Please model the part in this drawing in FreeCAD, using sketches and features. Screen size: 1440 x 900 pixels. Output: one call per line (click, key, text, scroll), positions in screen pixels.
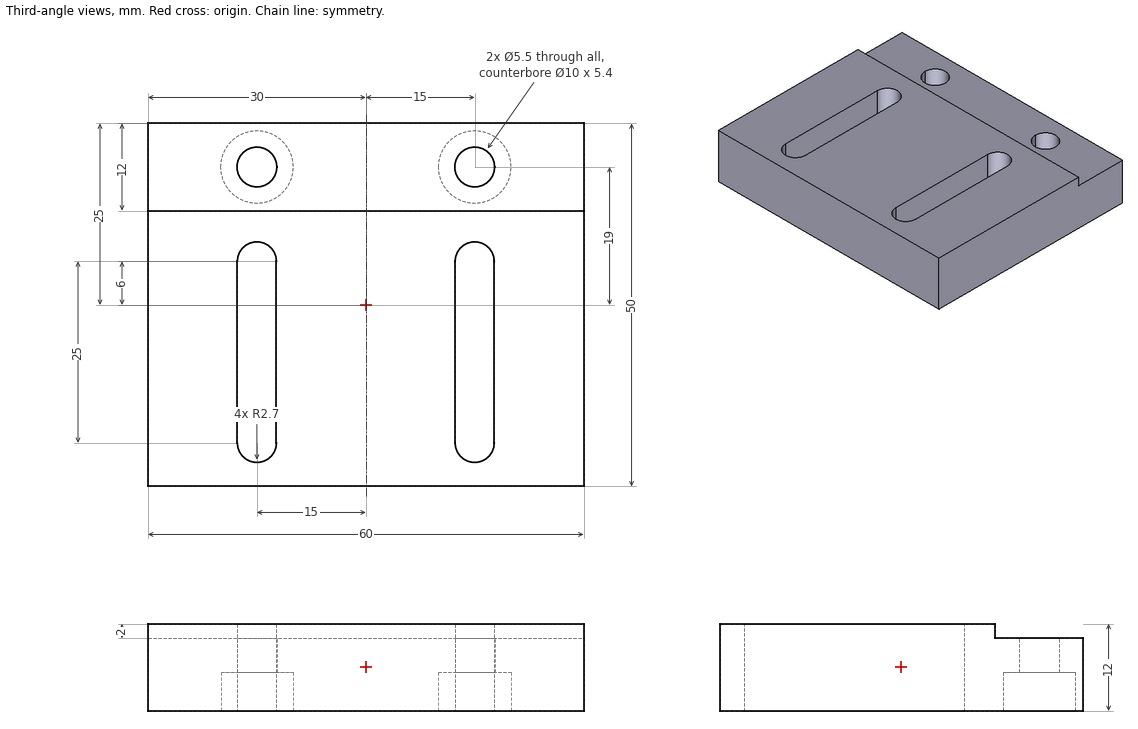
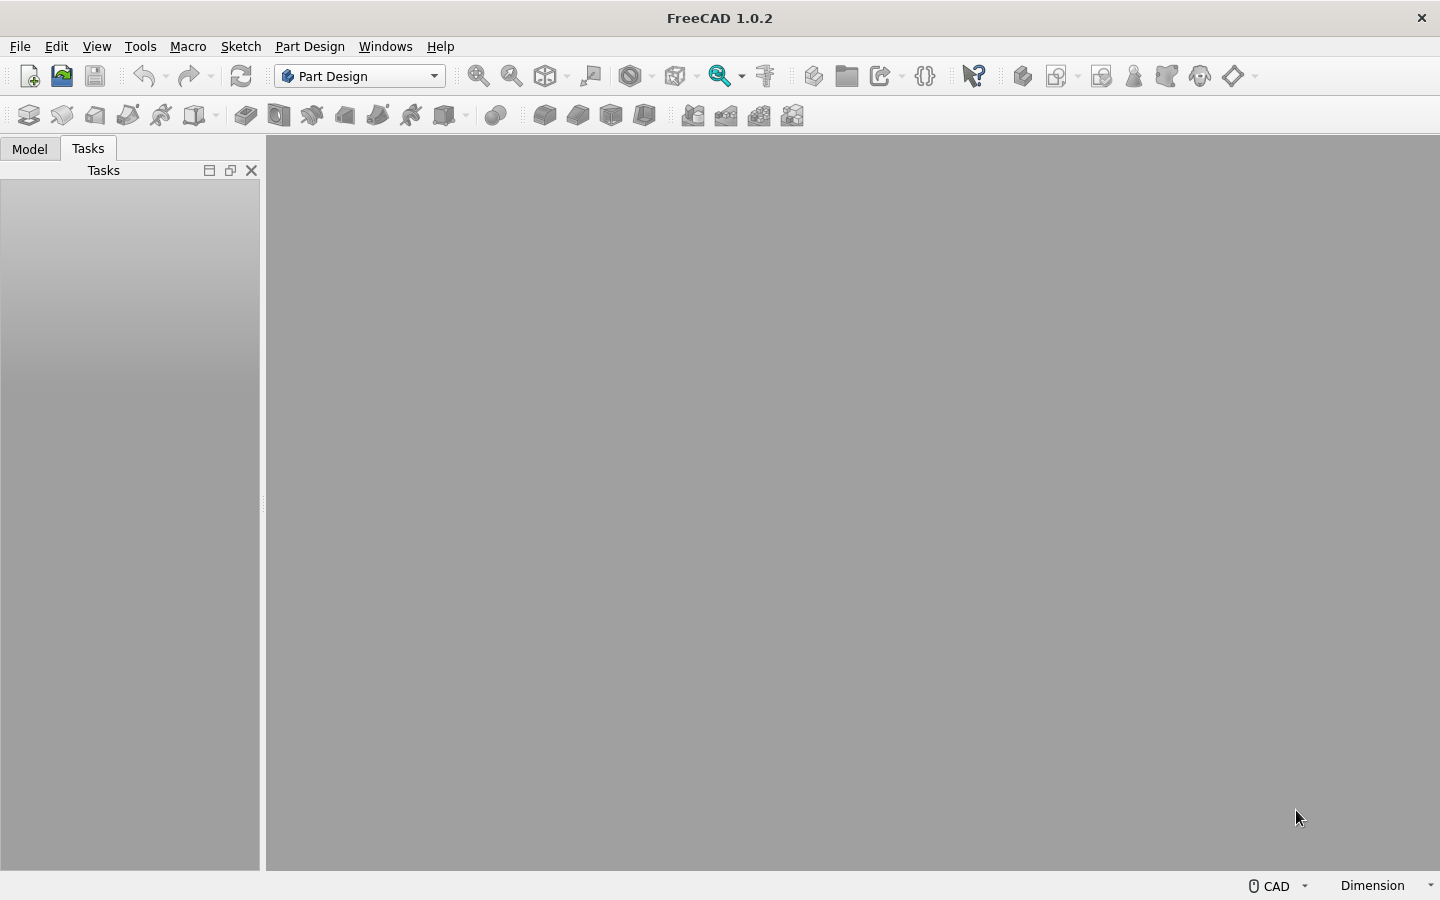
key(ctrl+n)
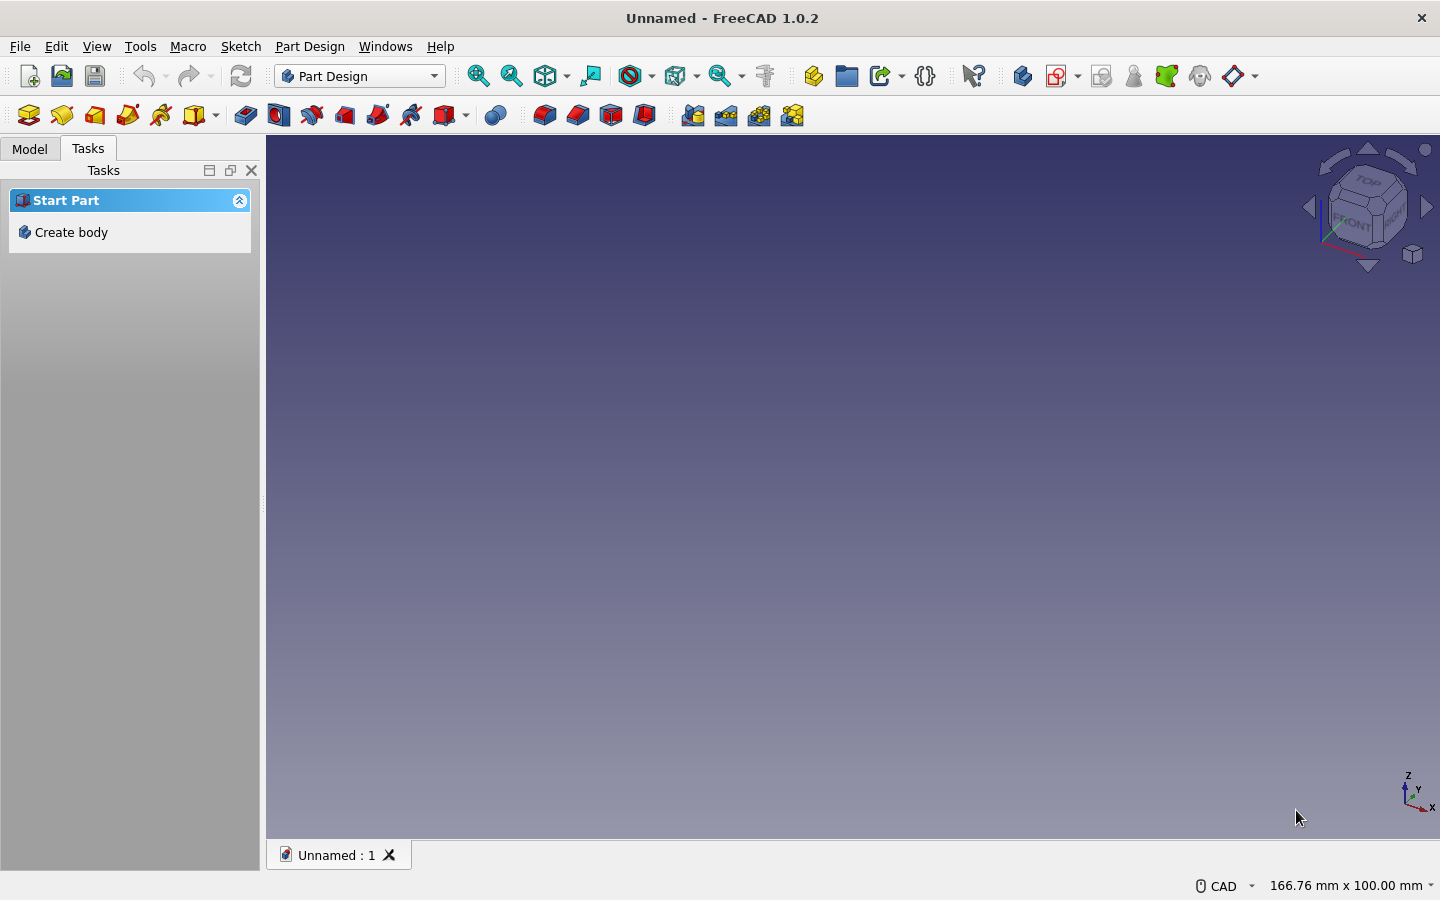
click(1056, 76)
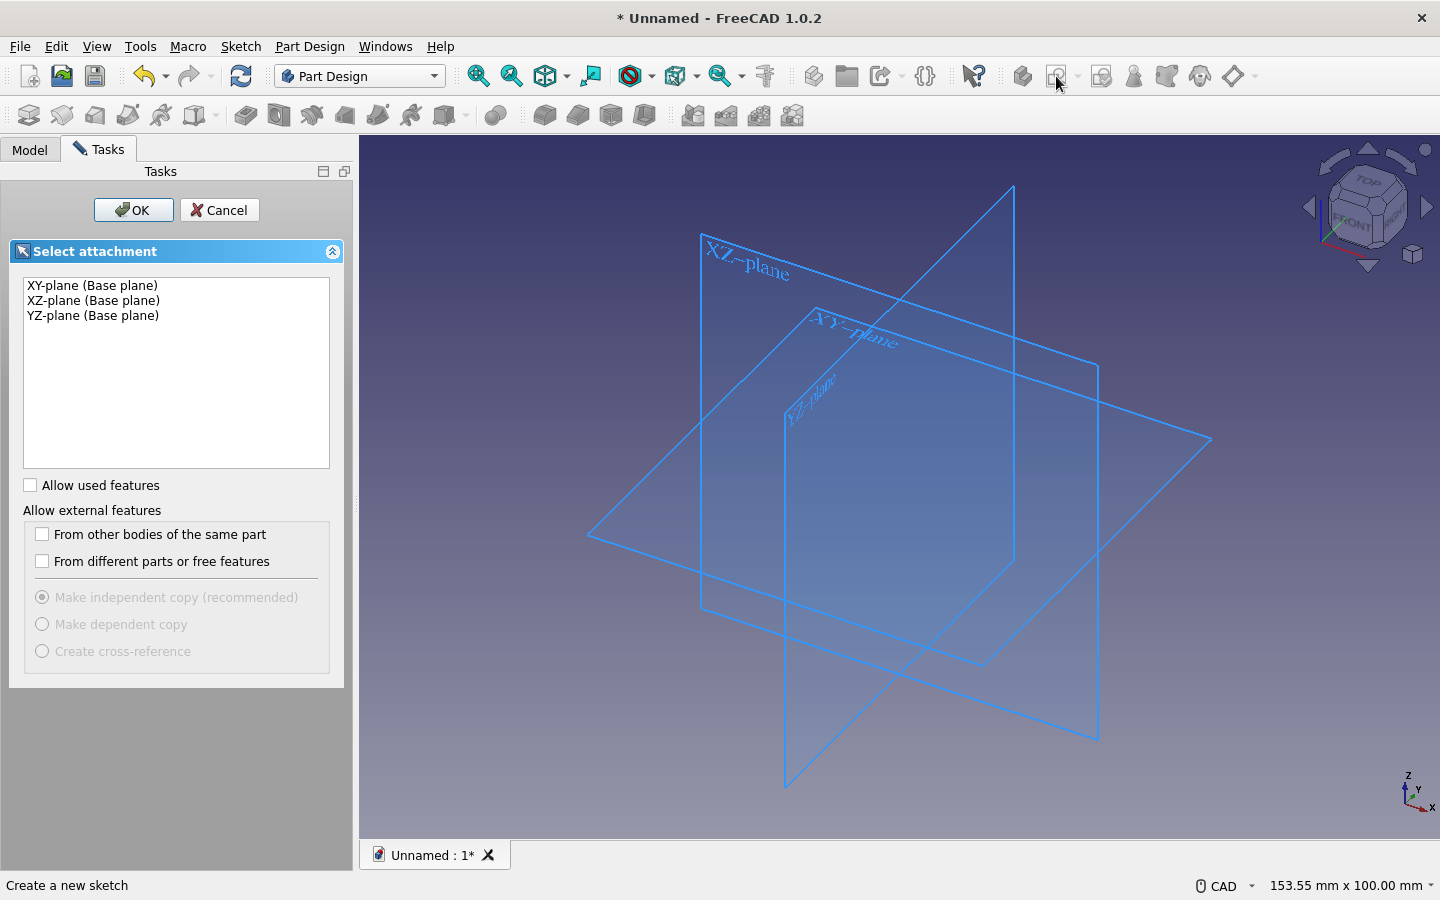
click(84, 286)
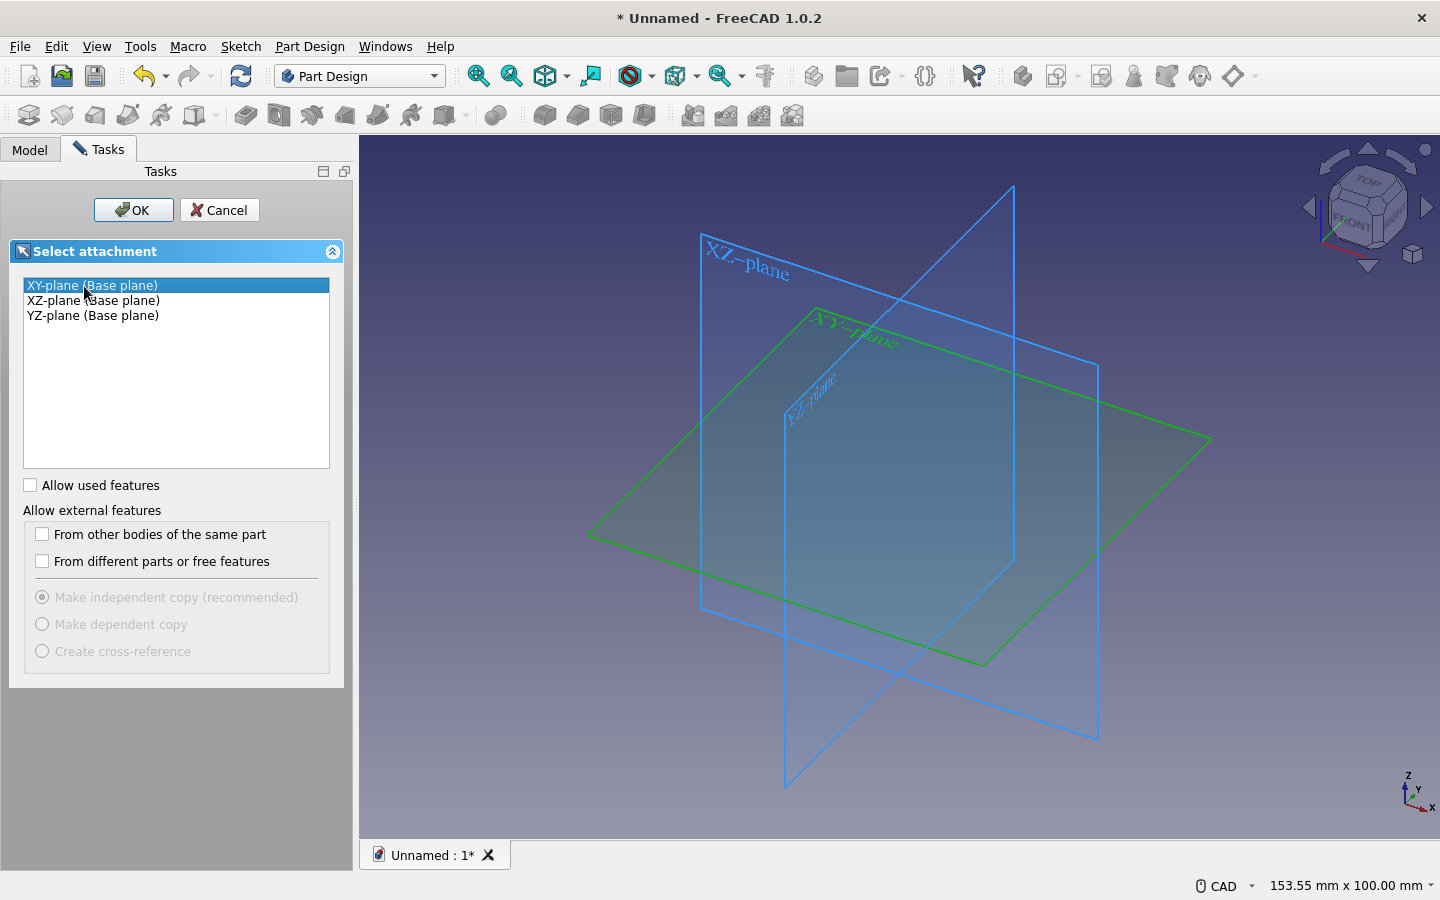
click(134, 210)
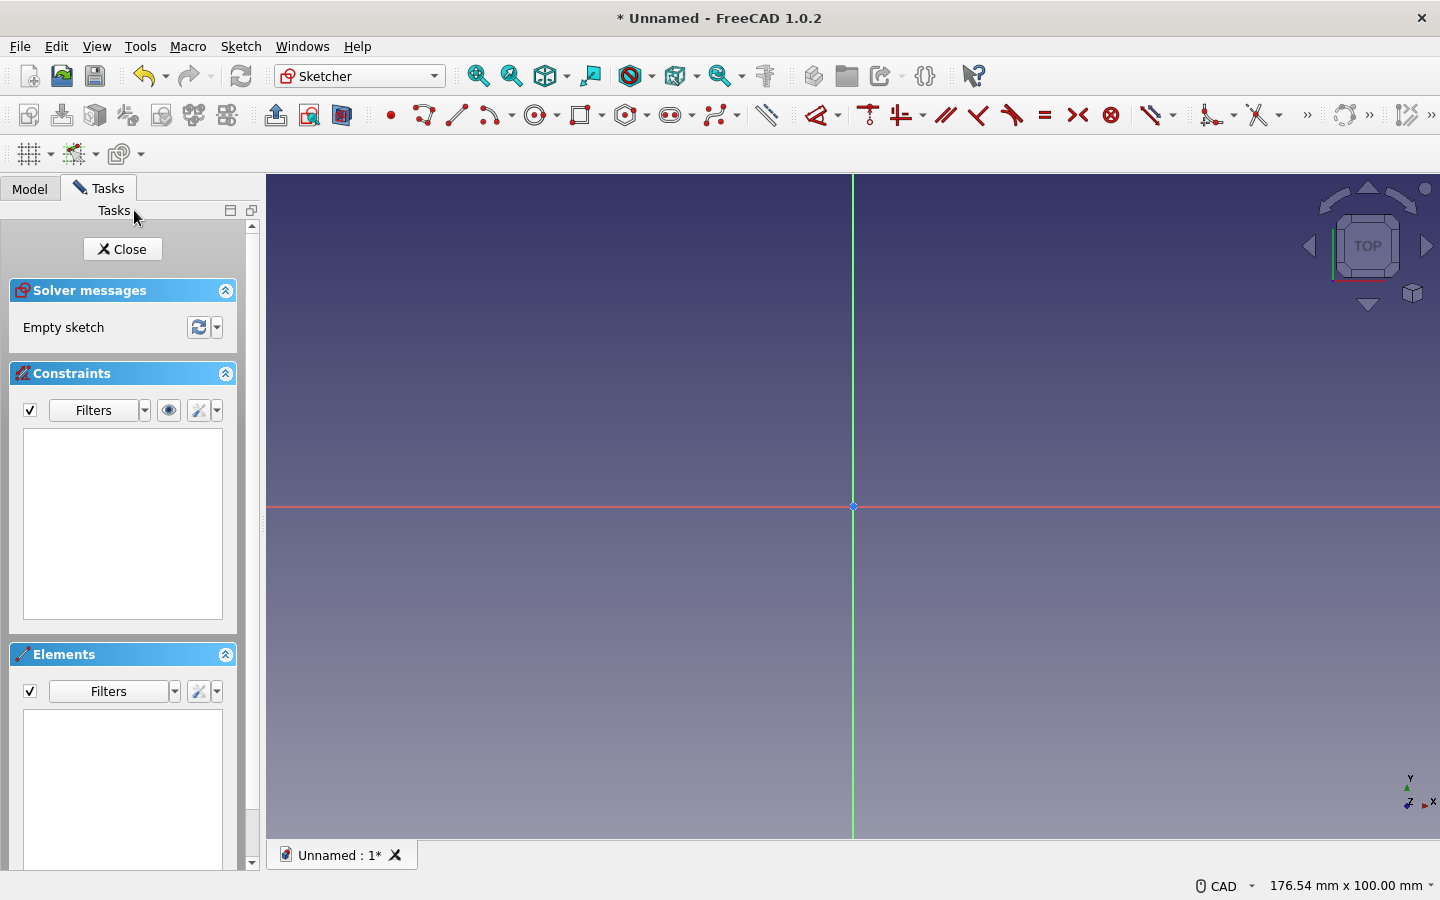
key(g)
key(v)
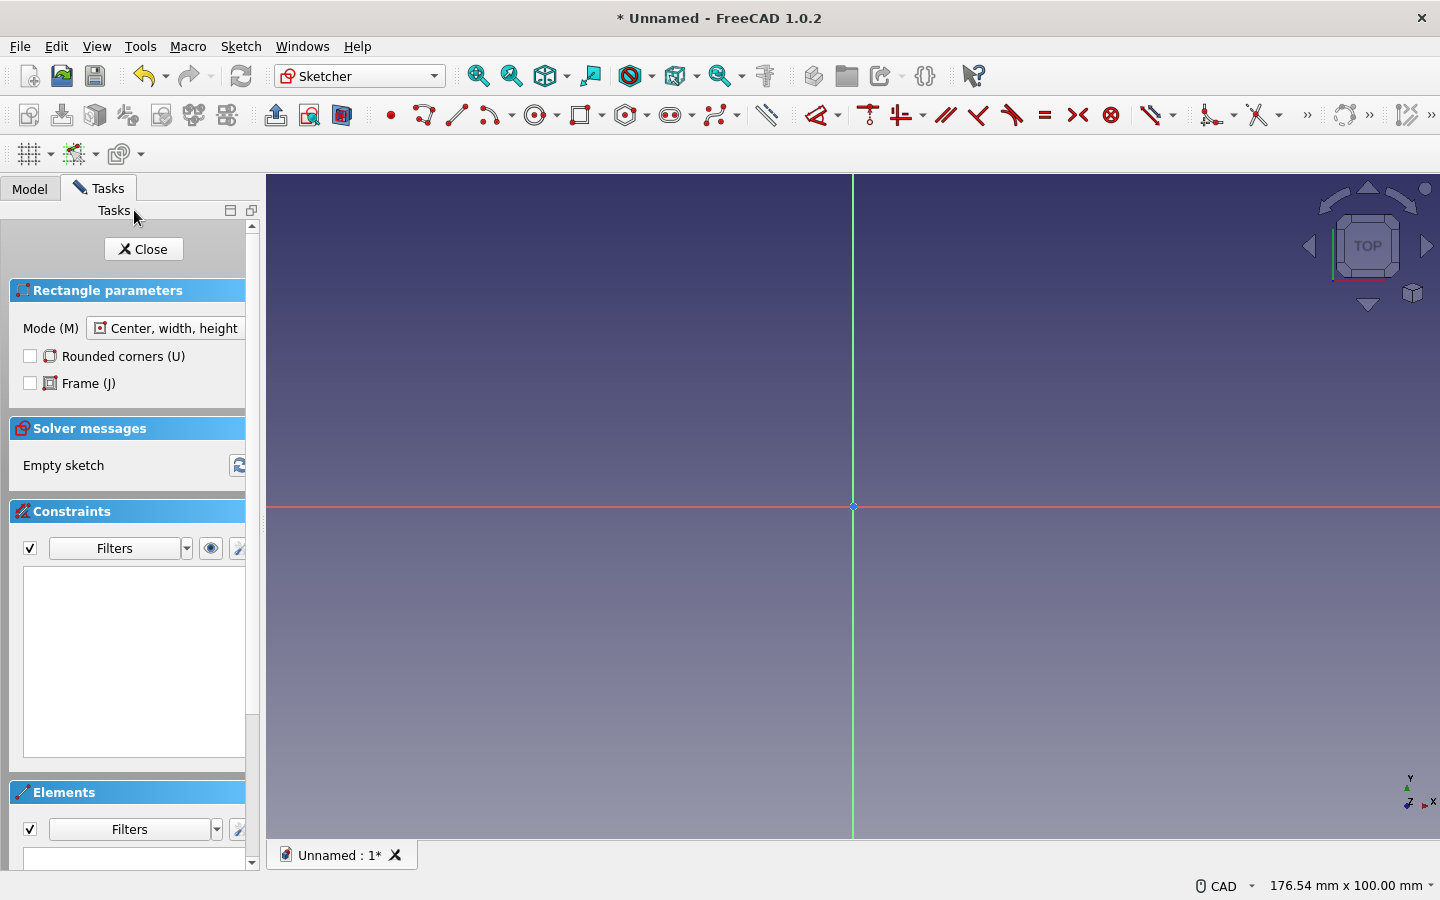
click(853, 506)
click(1052, 340)
key(Escape)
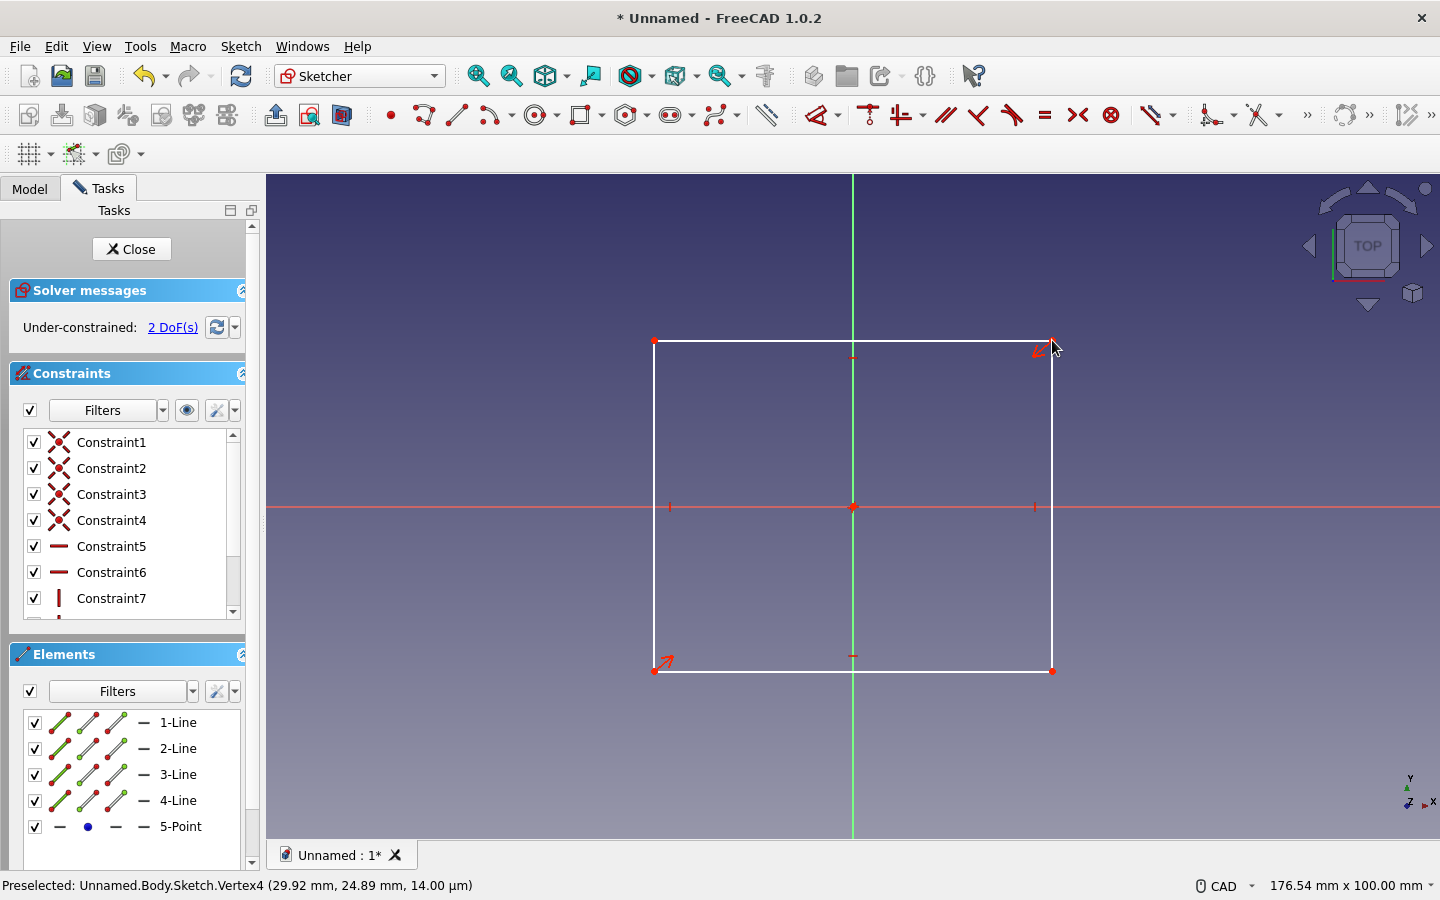
click(773, 672)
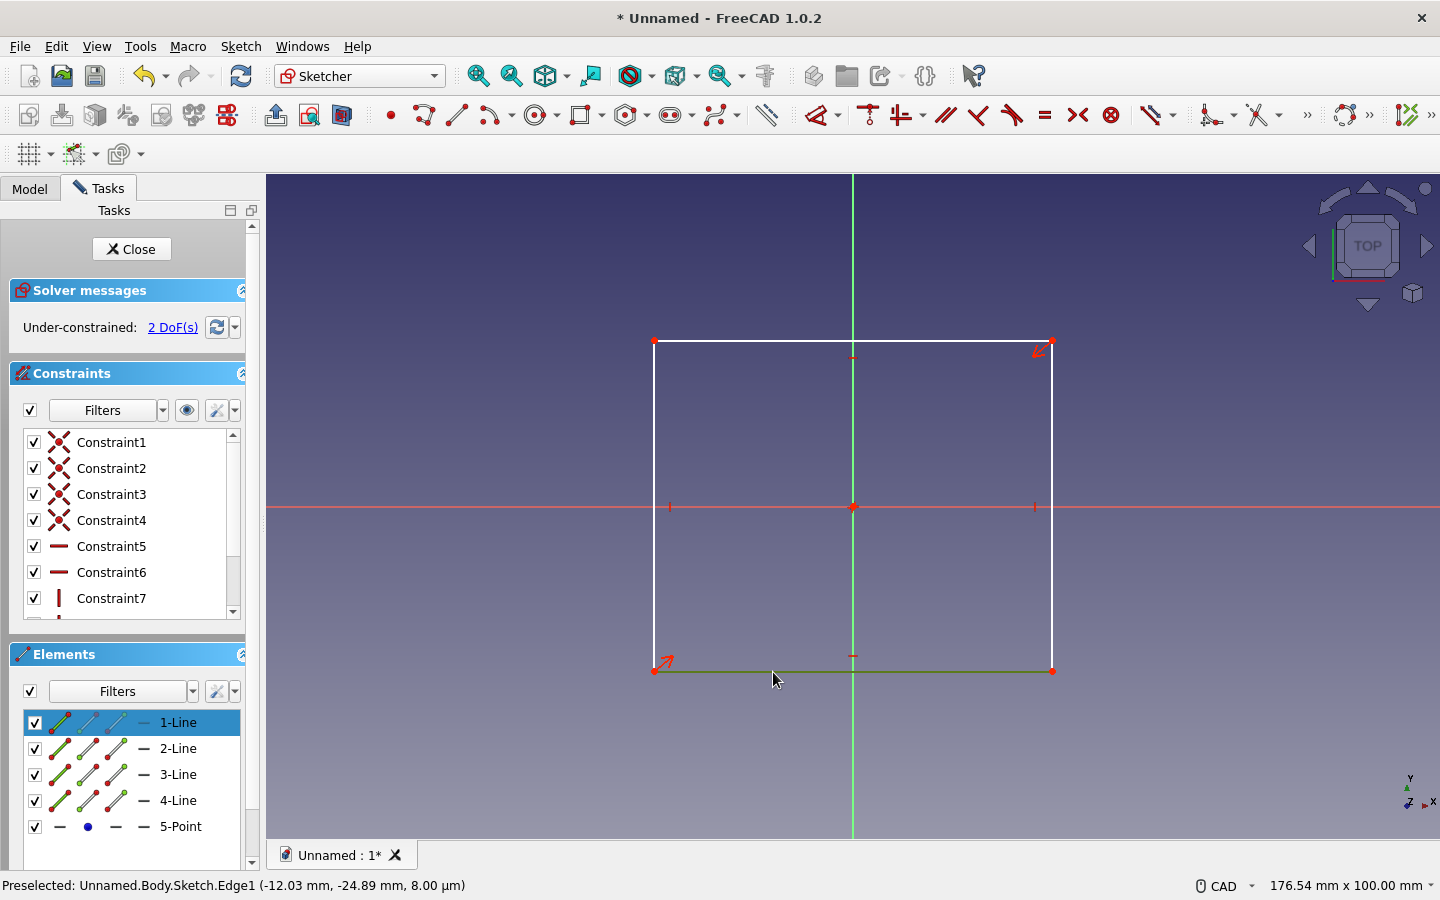
key(l)